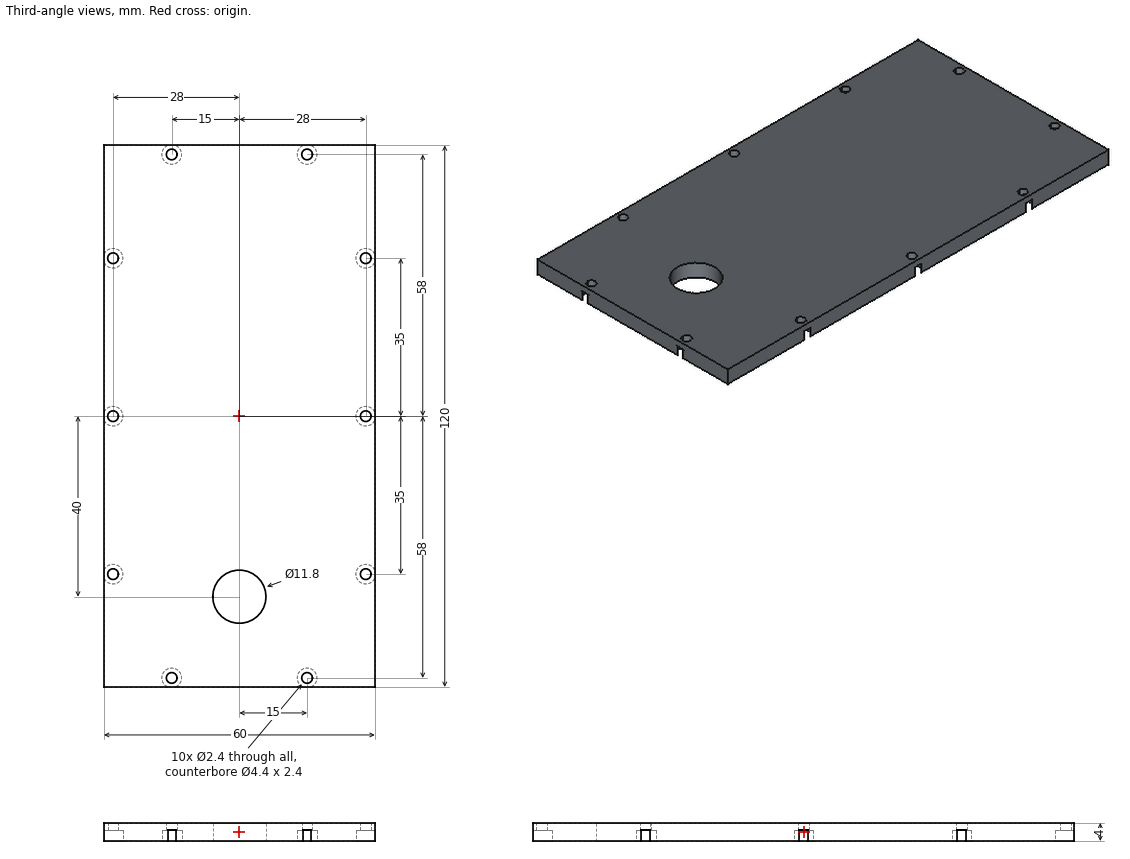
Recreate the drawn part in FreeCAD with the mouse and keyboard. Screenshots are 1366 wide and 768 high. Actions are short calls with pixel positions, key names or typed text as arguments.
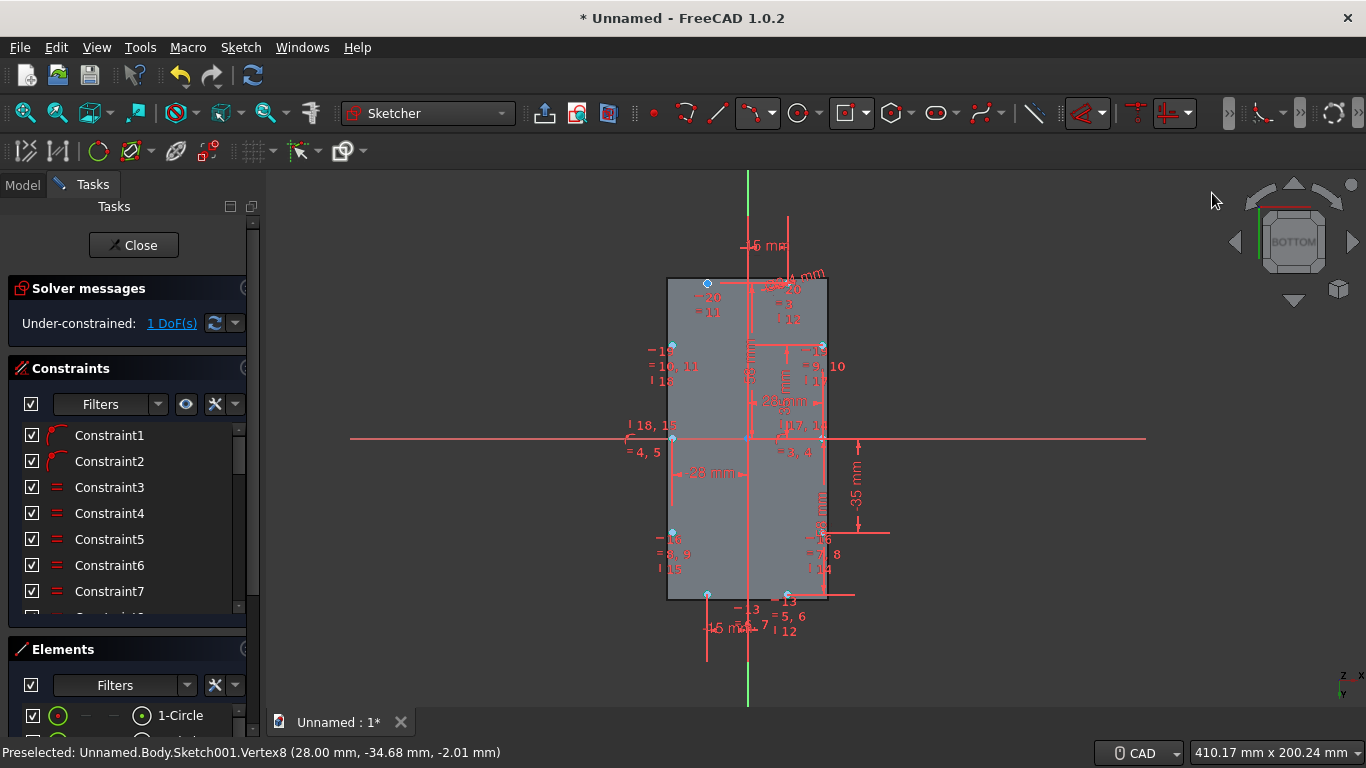
click(707, 283)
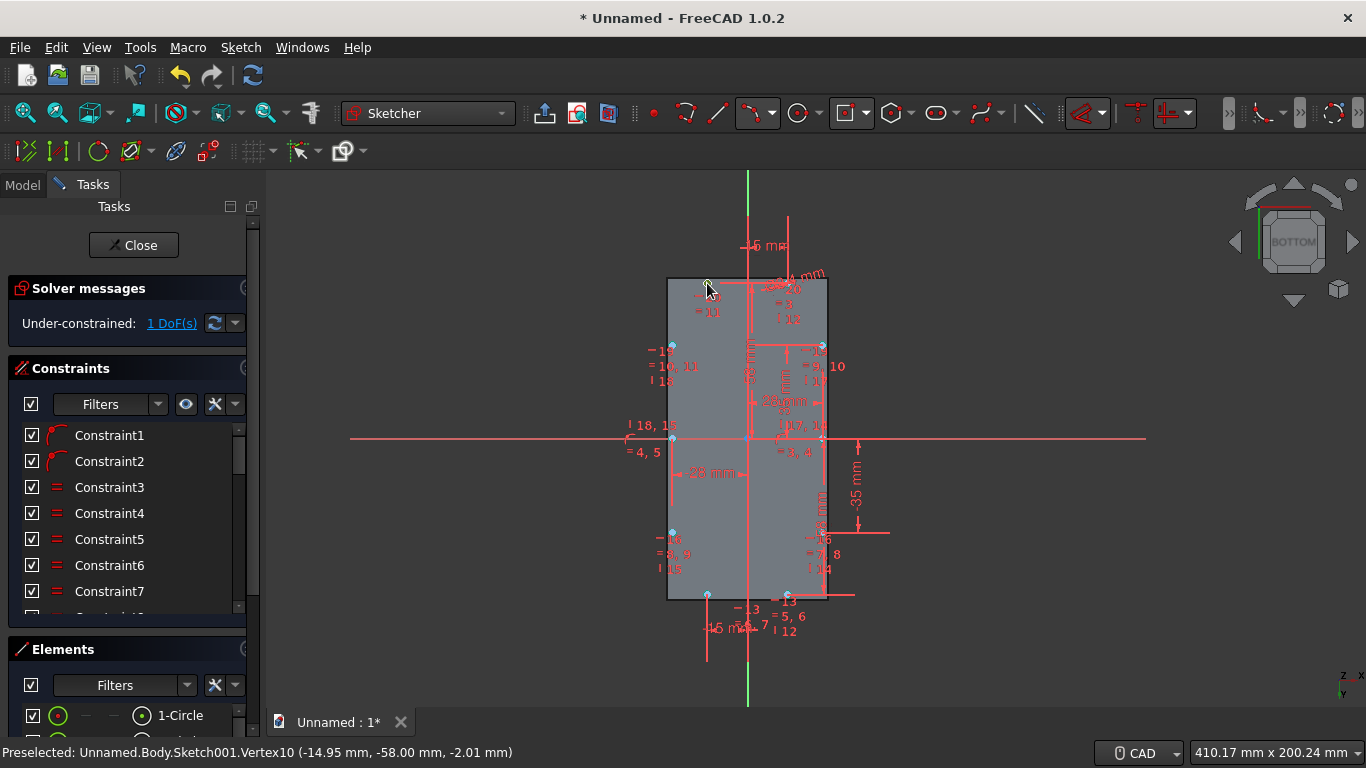
click(1104, 114)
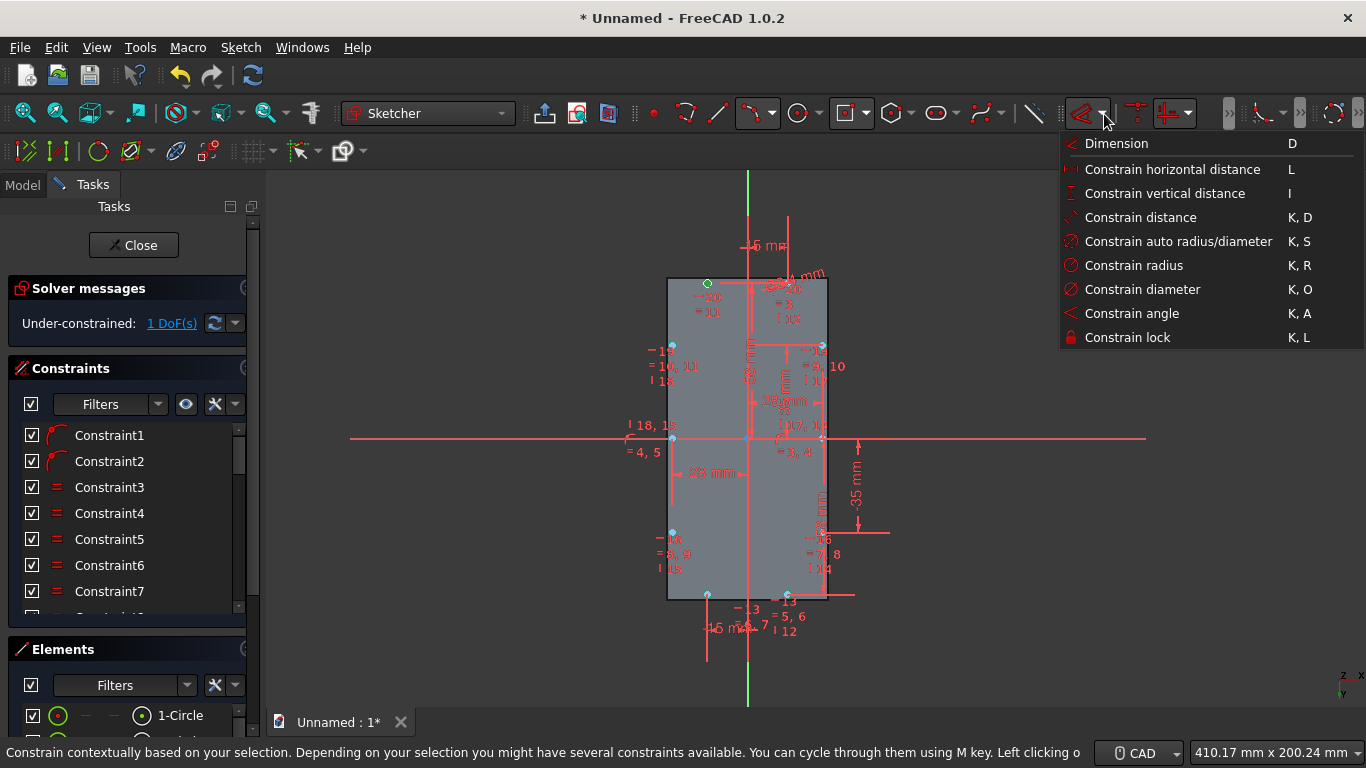
click(1212, 169)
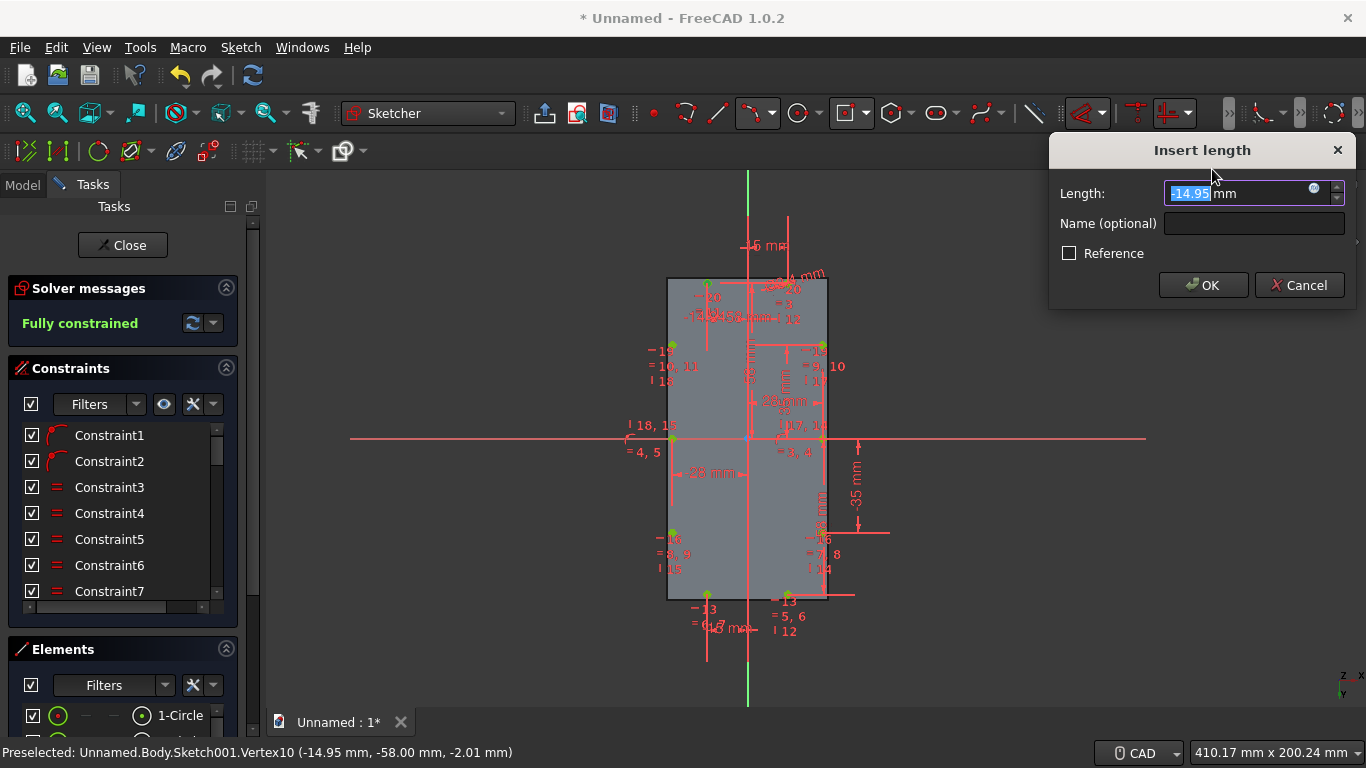
text(-15)
key(Return)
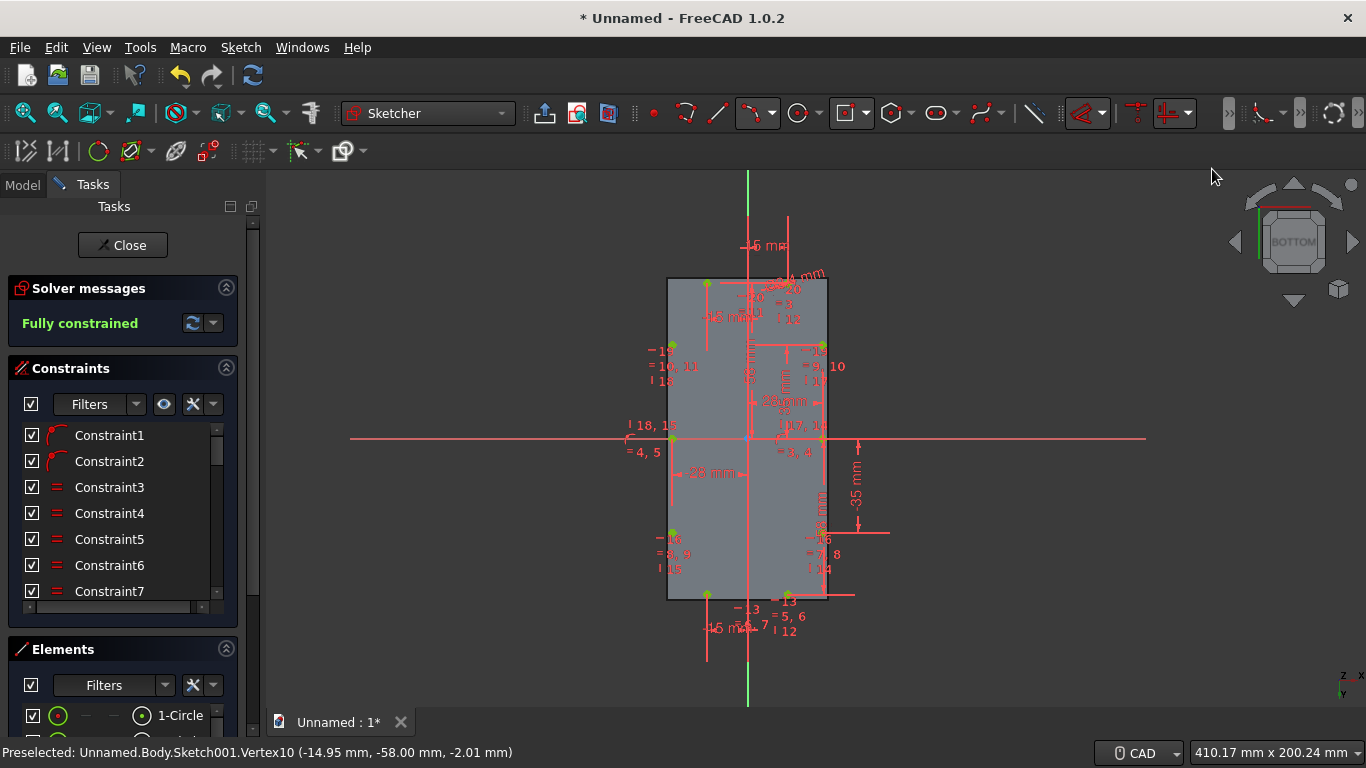
click(123, 245)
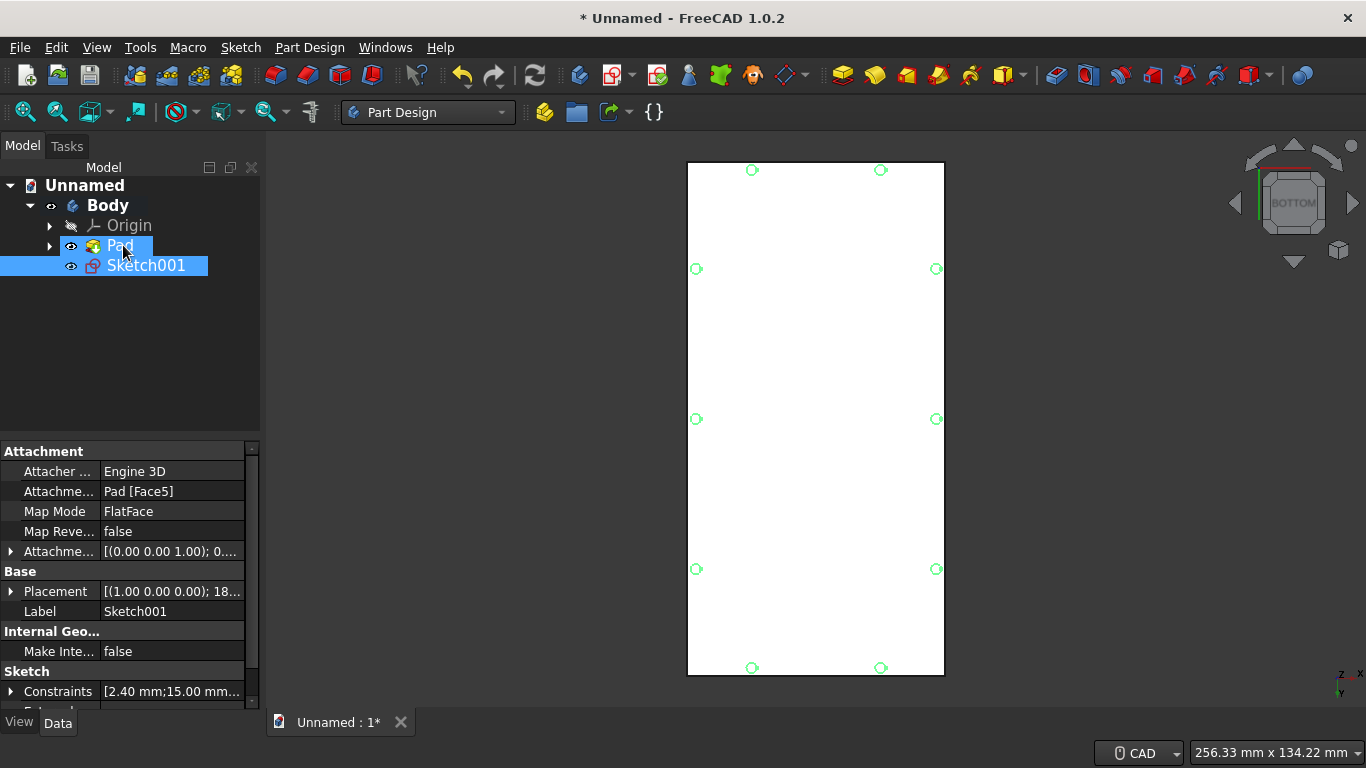
click(1090, 76)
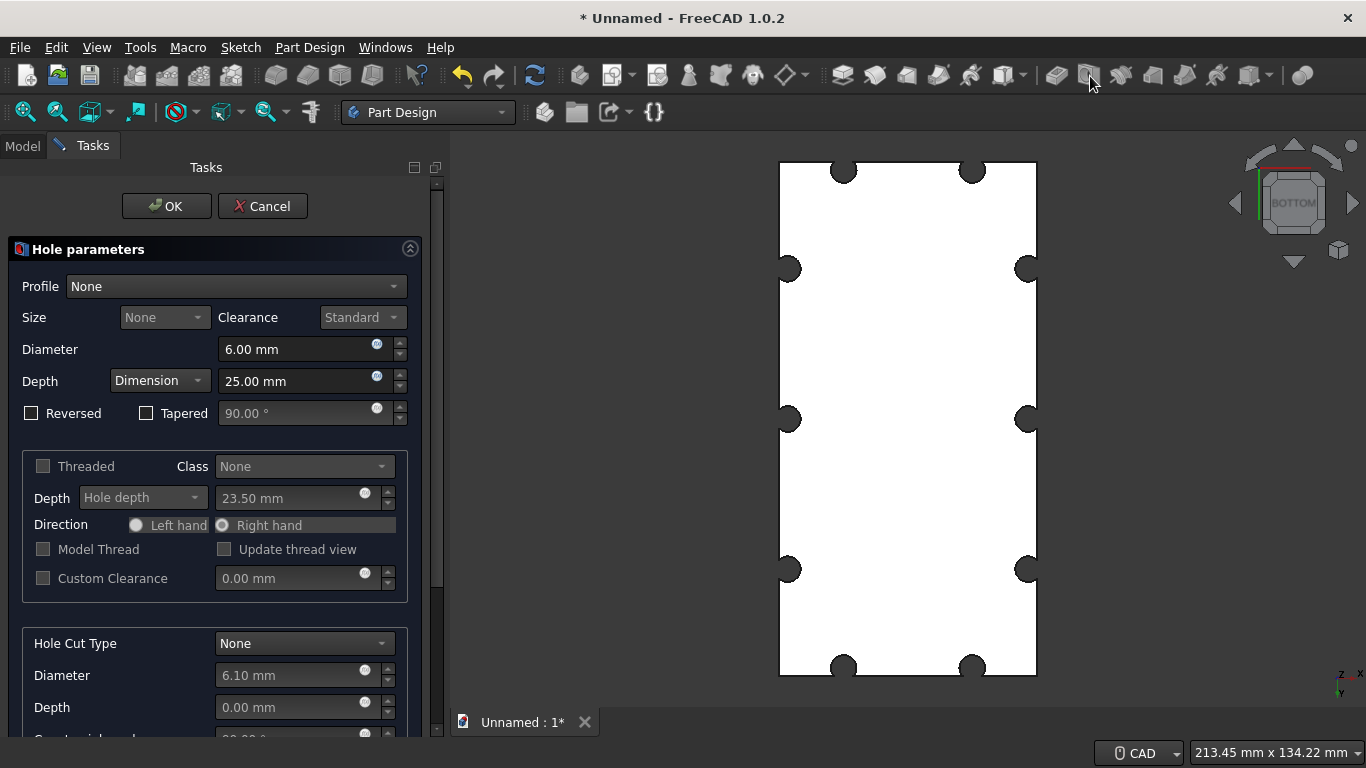
triple_click(305, 349)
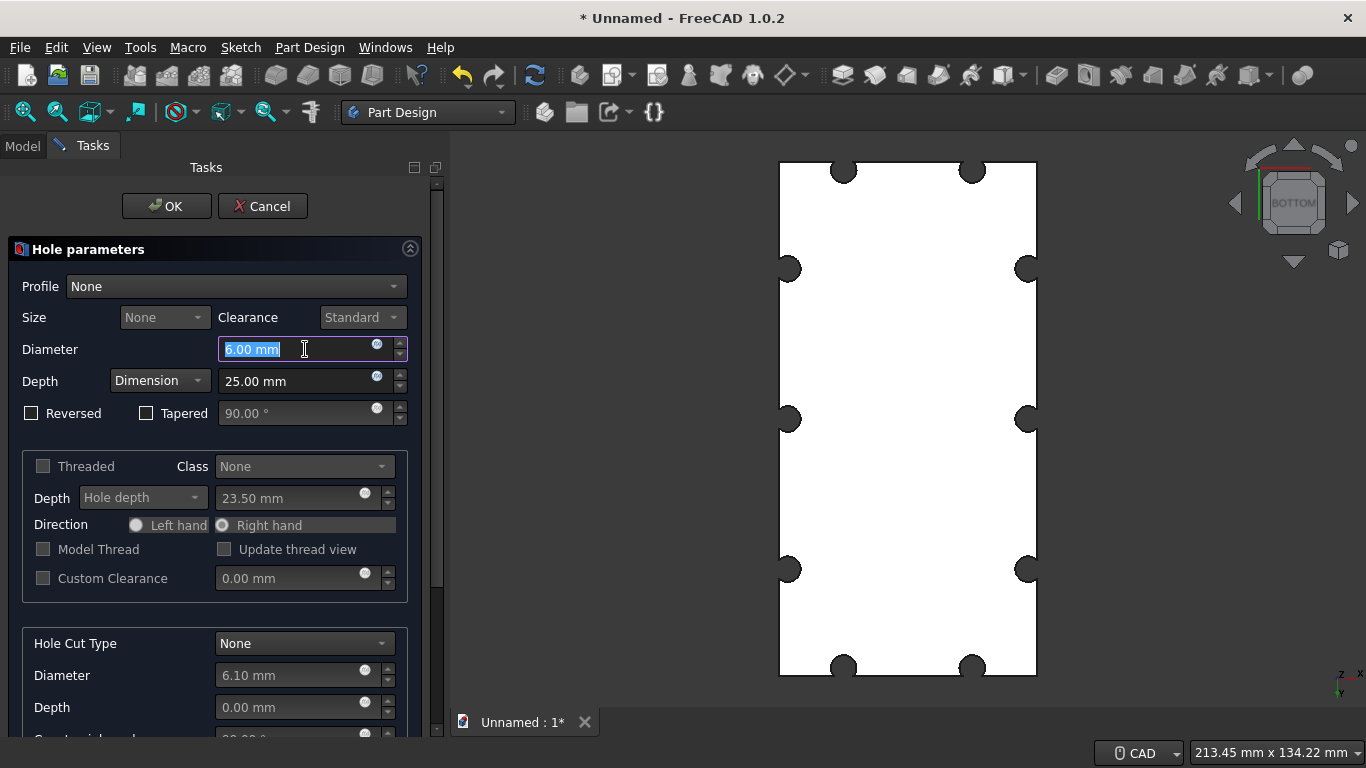
text(2.4)
key(Tab)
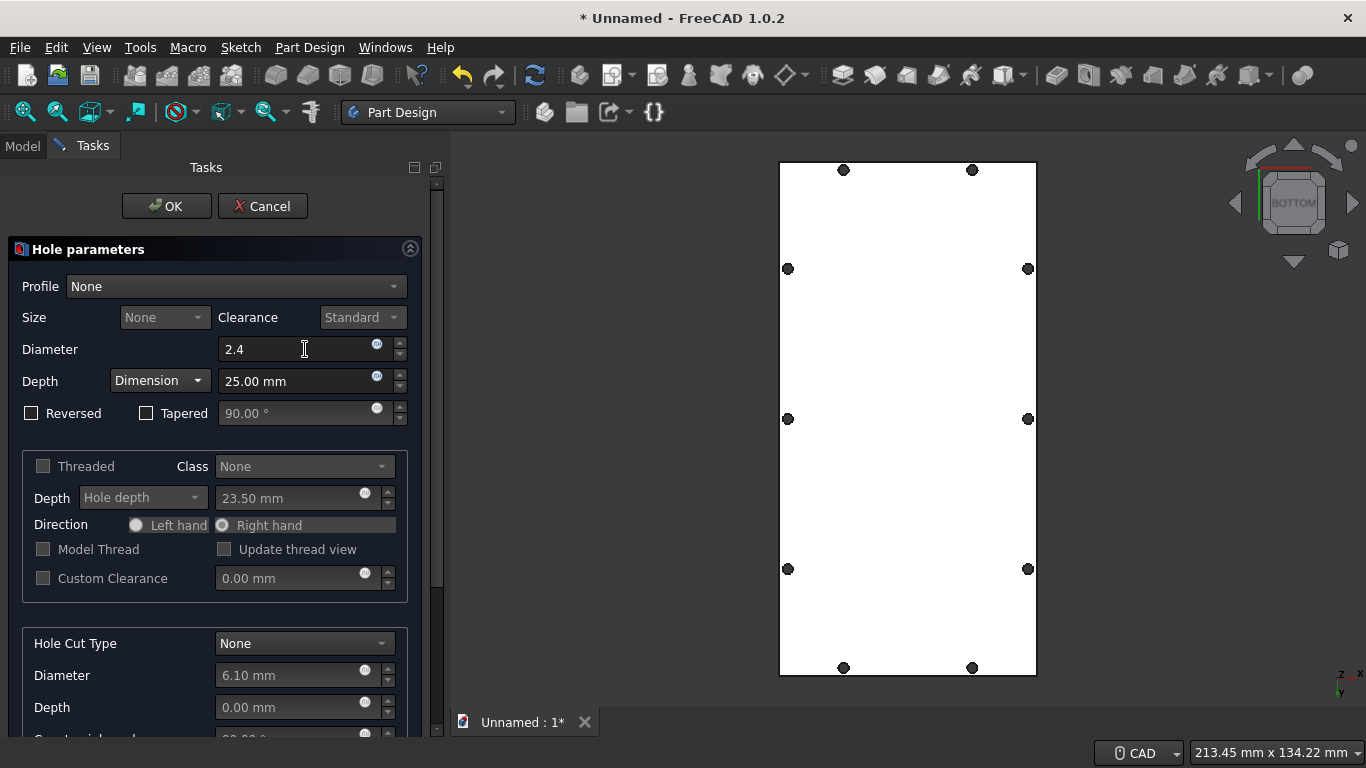
click(161, 380)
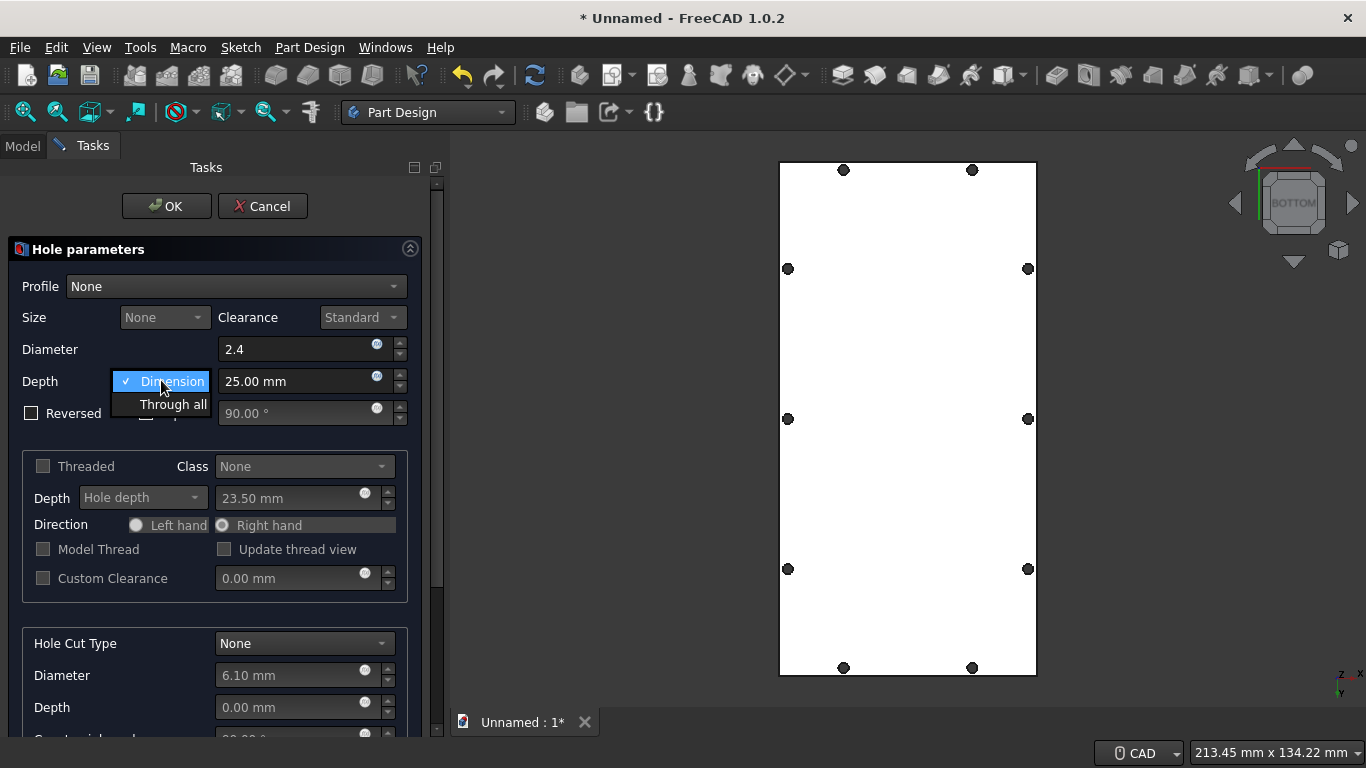
click(160, 404)